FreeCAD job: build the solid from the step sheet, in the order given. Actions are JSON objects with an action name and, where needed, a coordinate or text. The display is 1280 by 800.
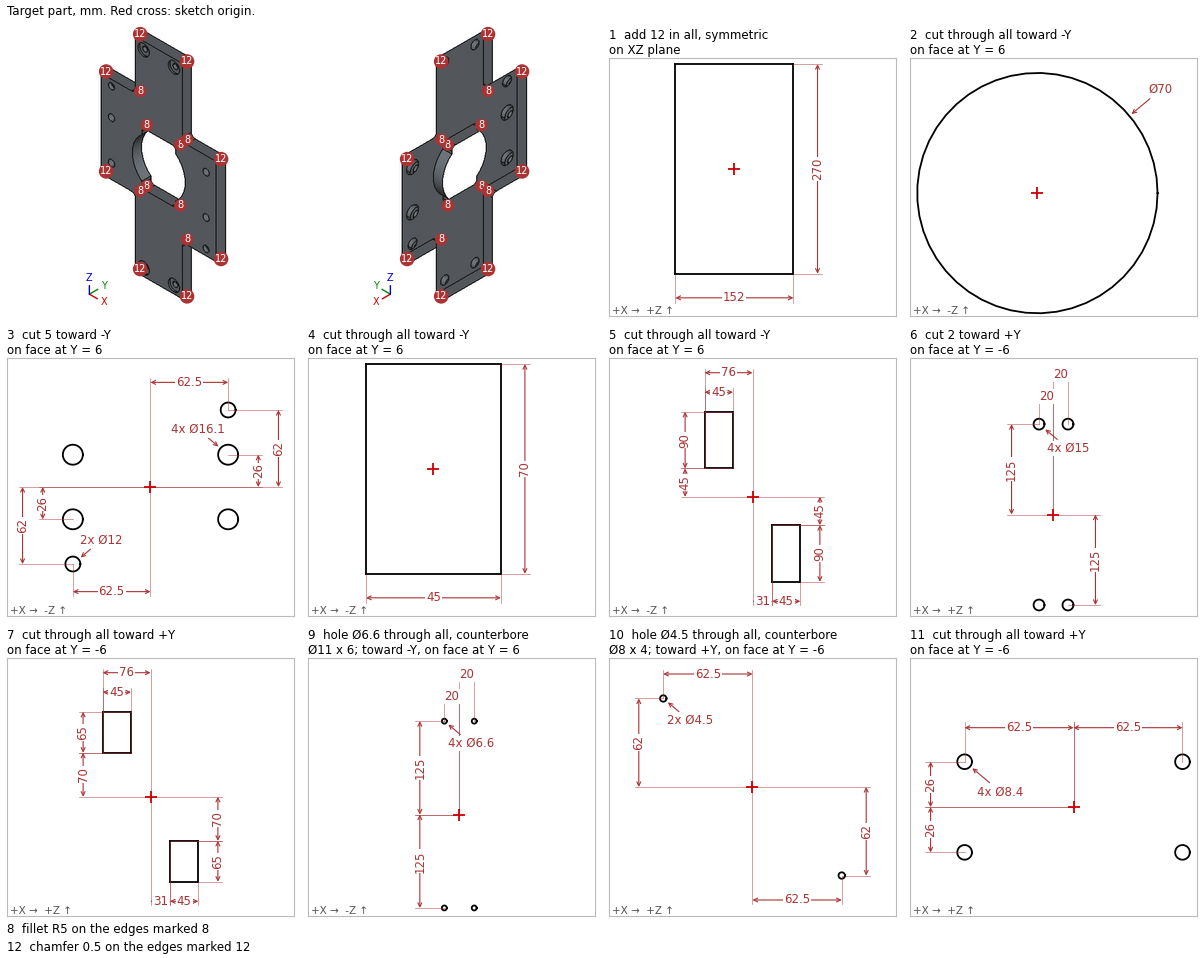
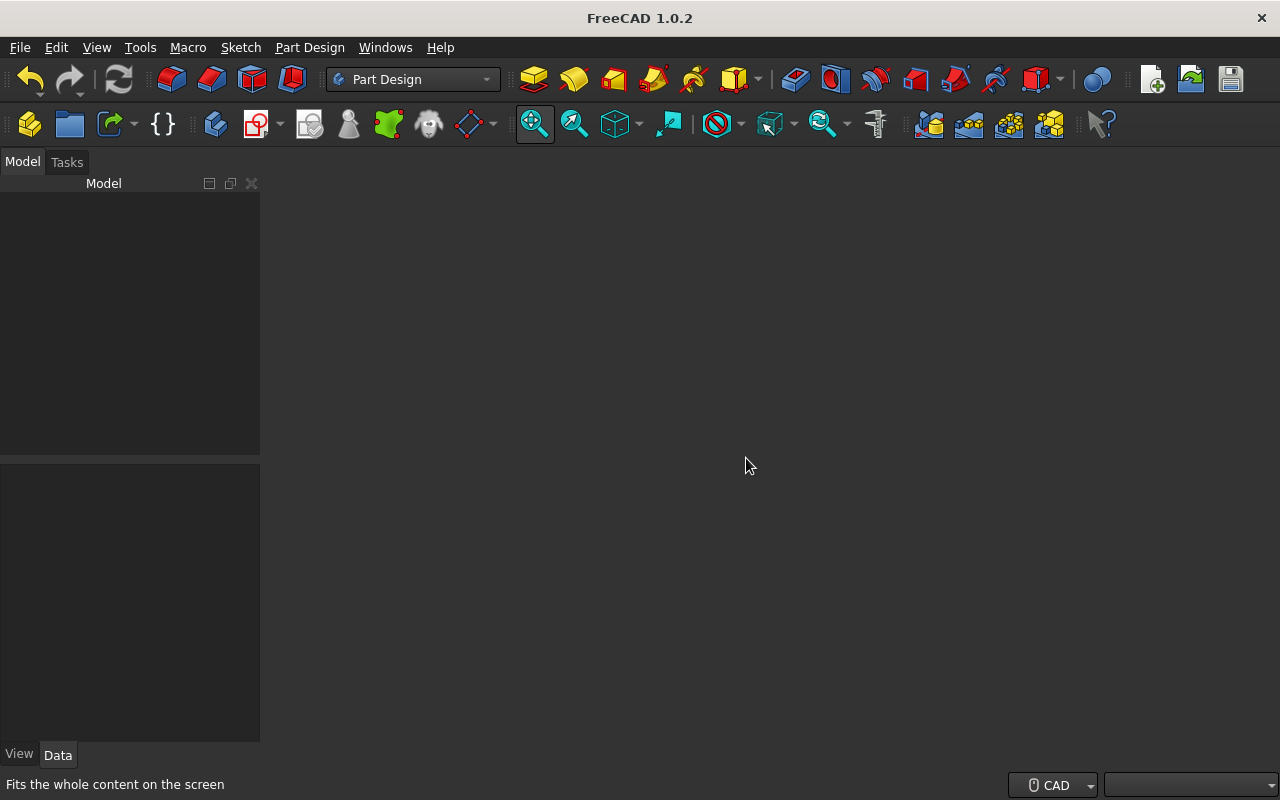
{"action": "left_click", "coordinate": [1152, 80]}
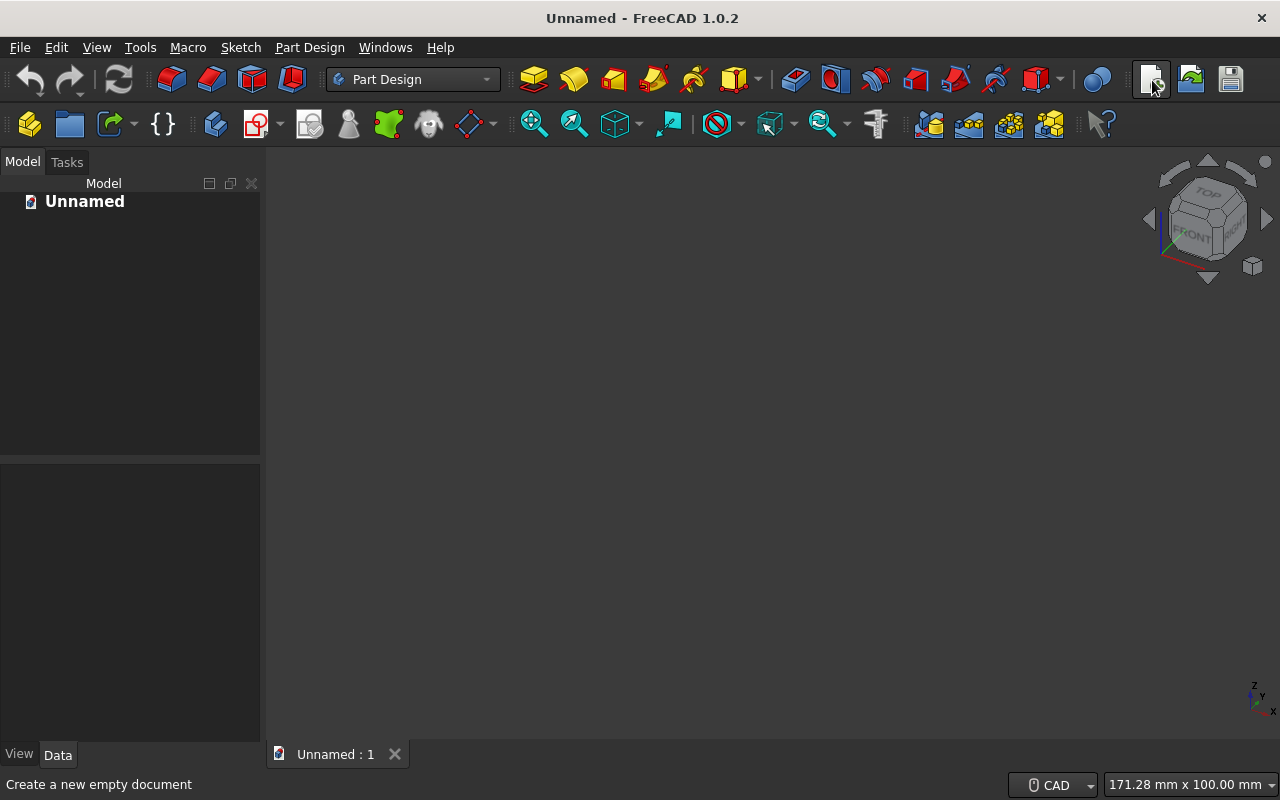
{"action": "left_click", "coordinate": [256, 124]}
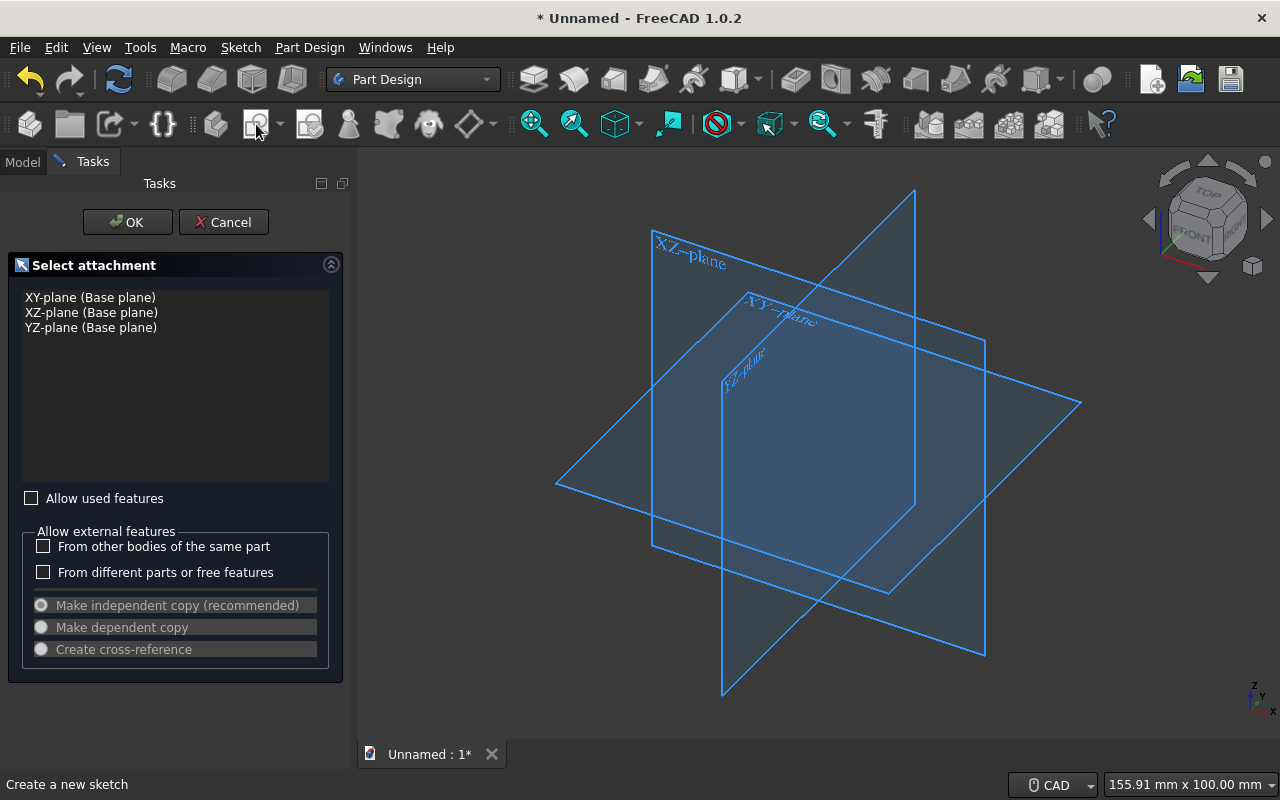
{"action": "left_click", "coordinate": [82, 312]}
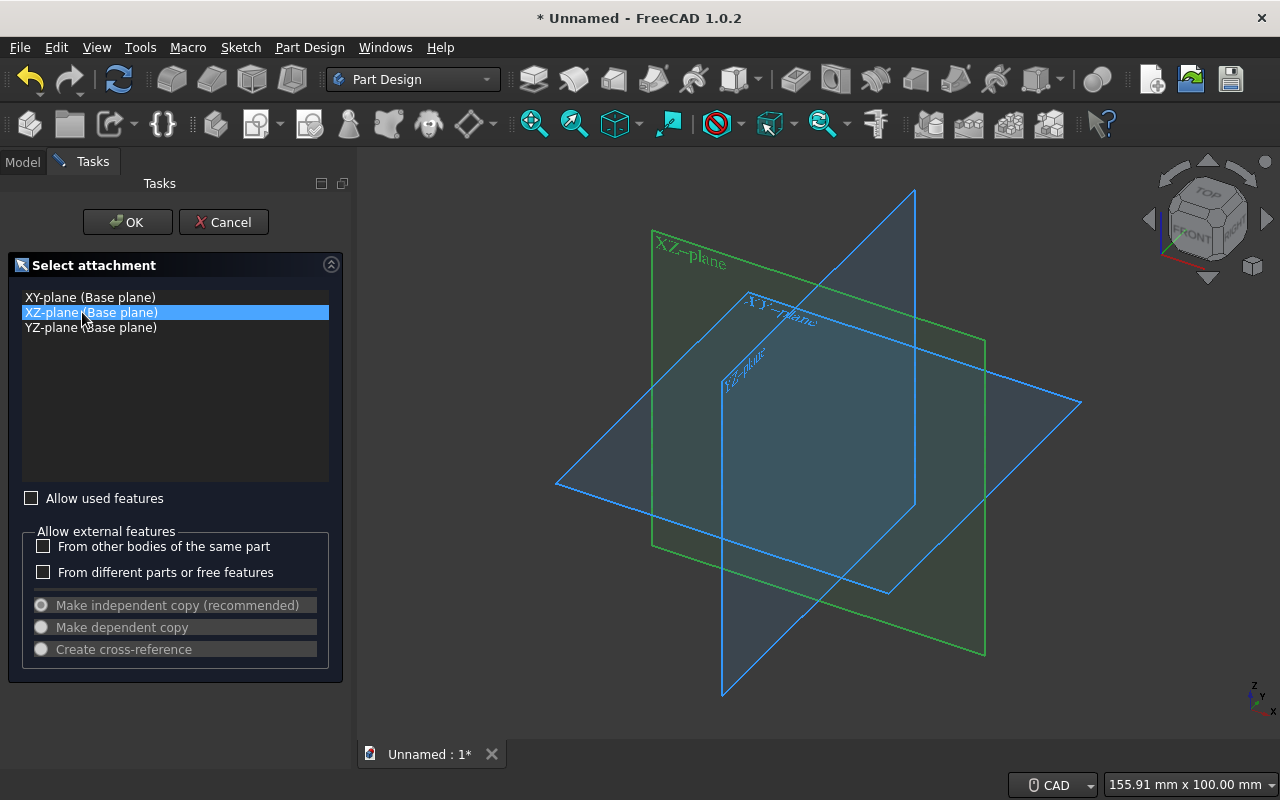
{"action": "left_click", "coordinate": [128, 222]}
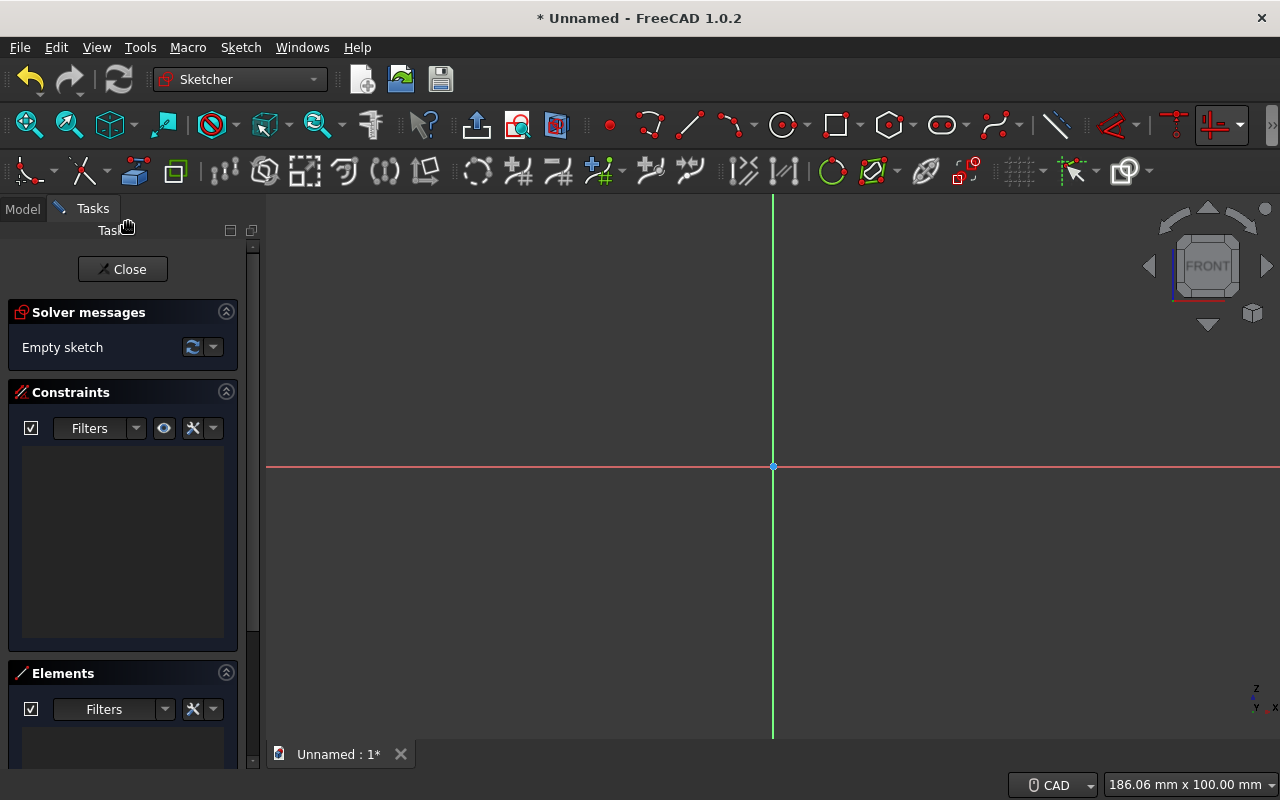
{"action": "scroll", "coordinate": [682, 466], "scroll_direction": "down", "scroll_amount": 7}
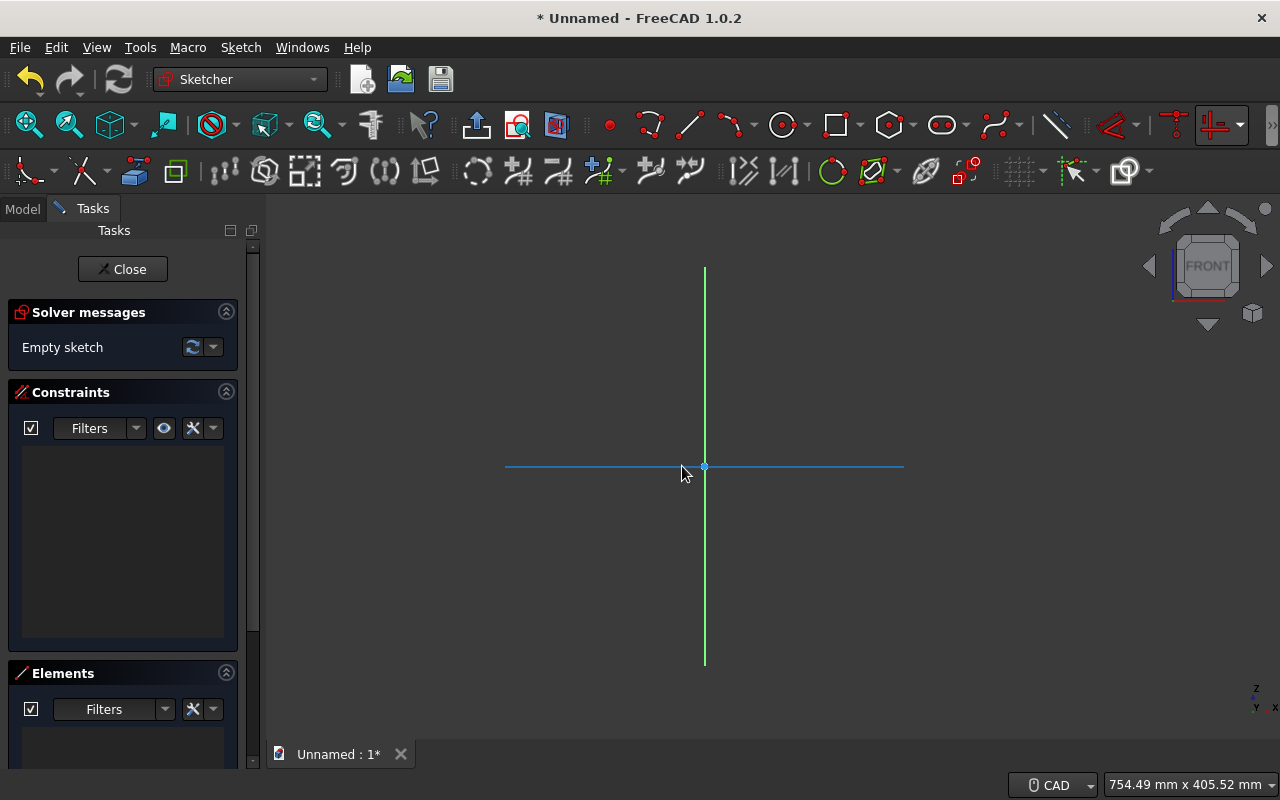
{"action": "key", "text": "g v"}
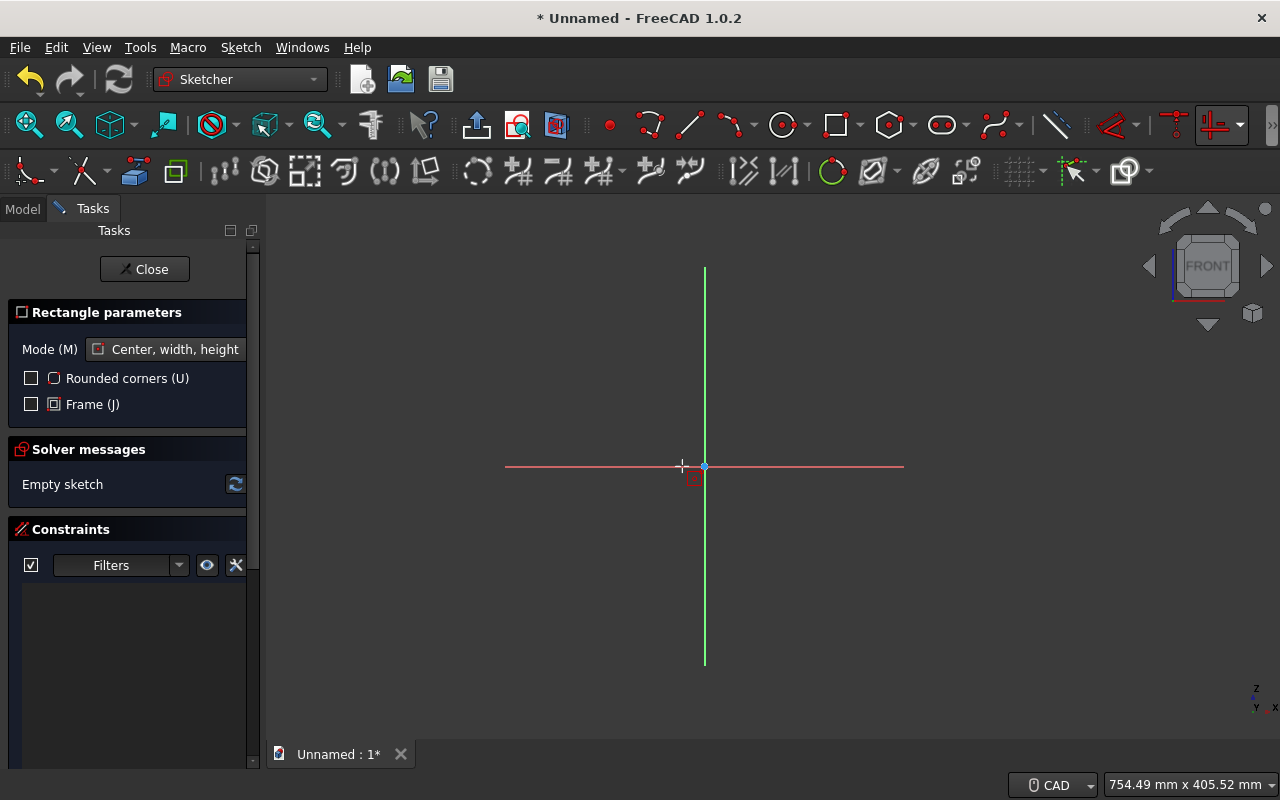
{"action": "left_click", "coordinate": [705, 466]}
{"action": "mouse_move", "coordinate": [807, 285]}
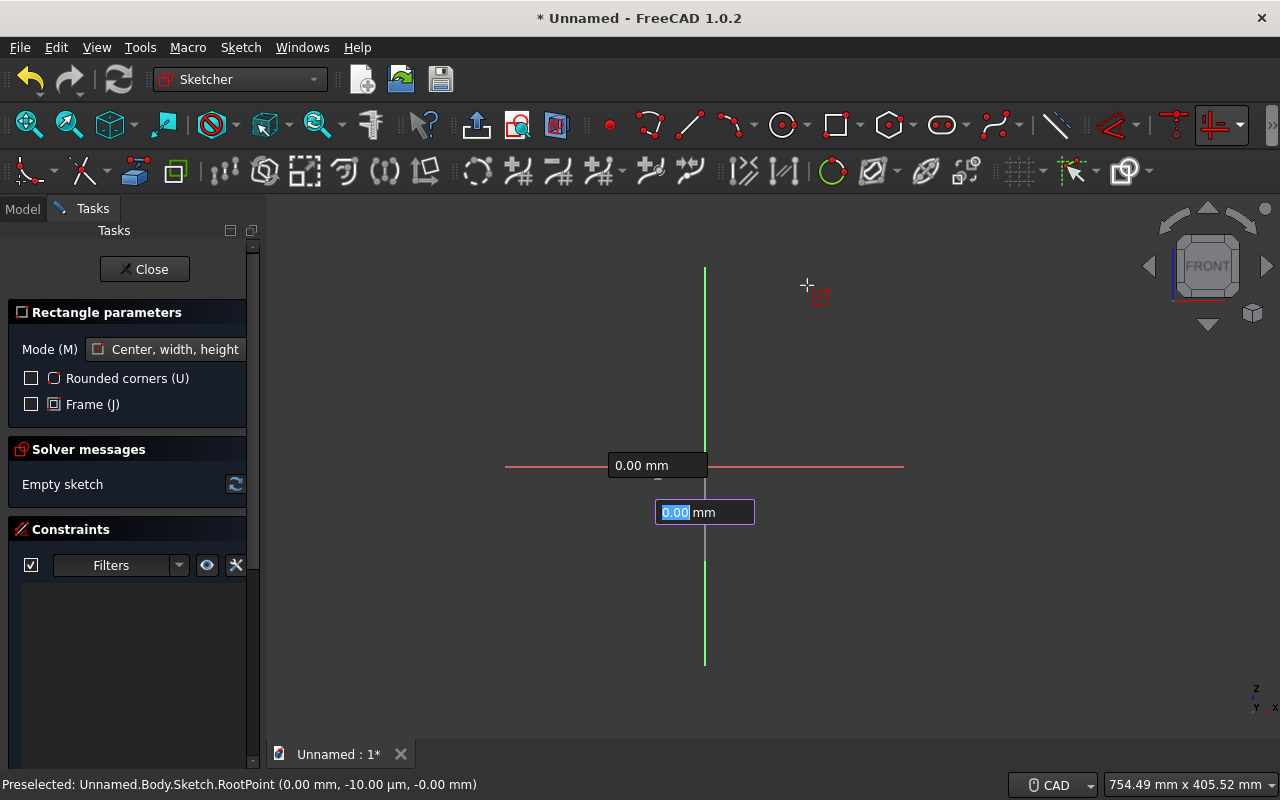
{"action": "type", "text": "152"}
{"action": "key", "text": "Tab"}
{"action": "type", "text": "270"}
{"action": "key", "text": "Return"}
{"action": "key", "text": "Escape"}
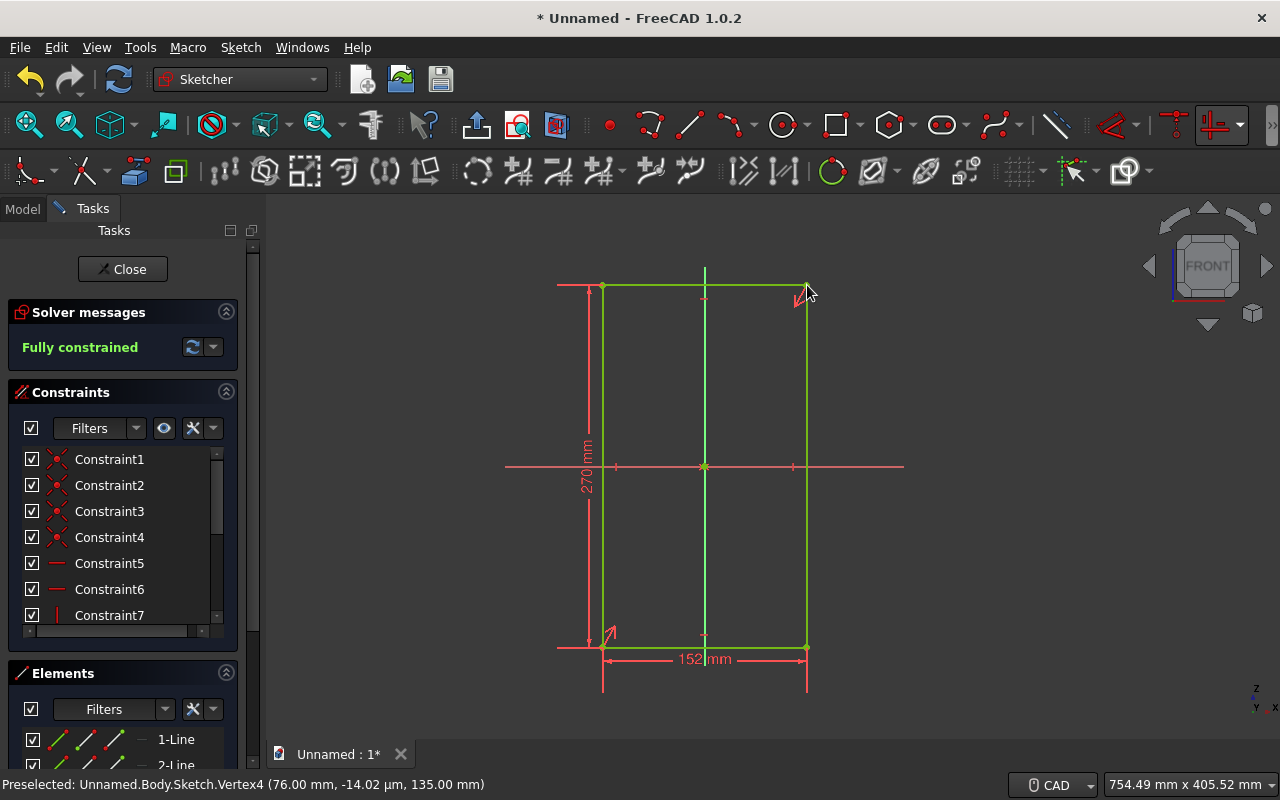
{"action": "left_click", "coordinate": [123, 269]}